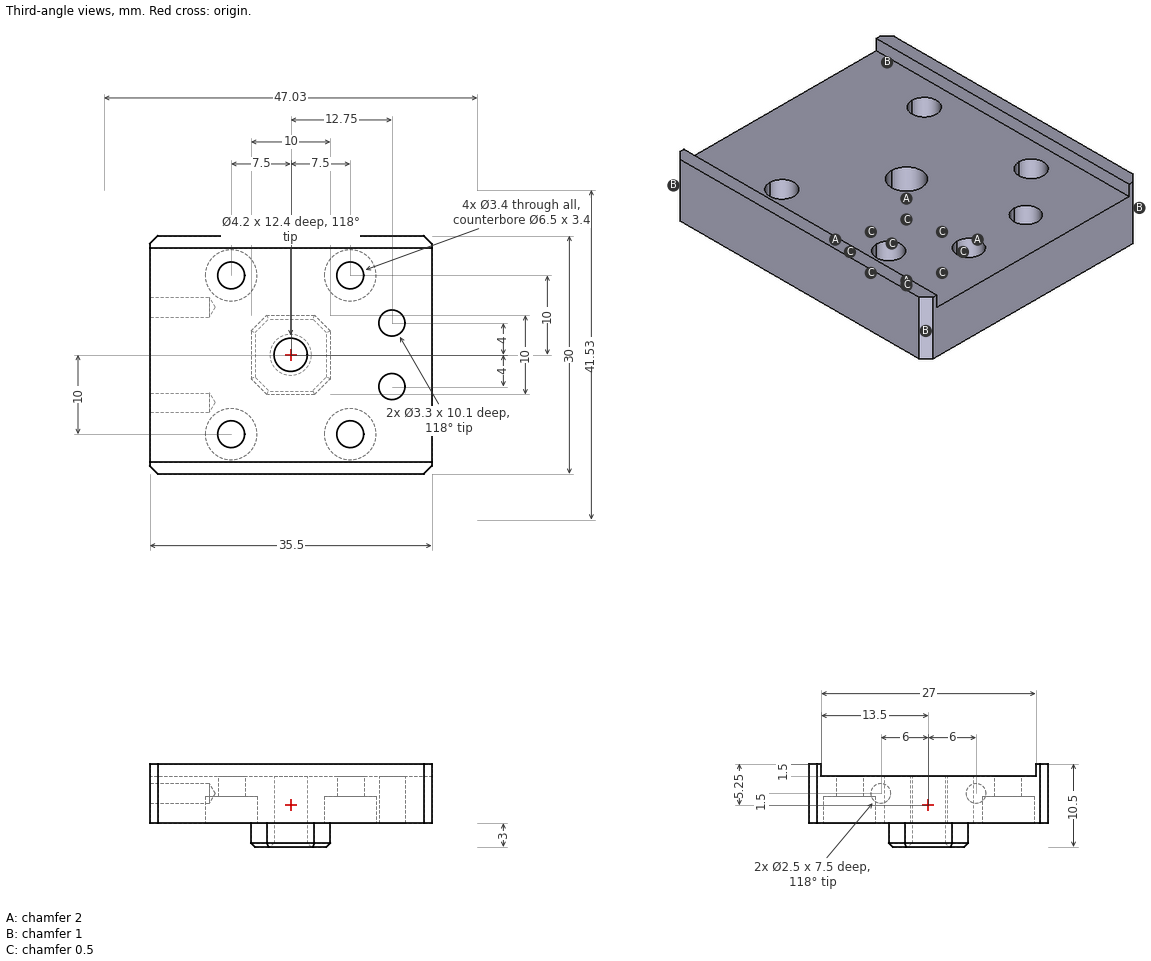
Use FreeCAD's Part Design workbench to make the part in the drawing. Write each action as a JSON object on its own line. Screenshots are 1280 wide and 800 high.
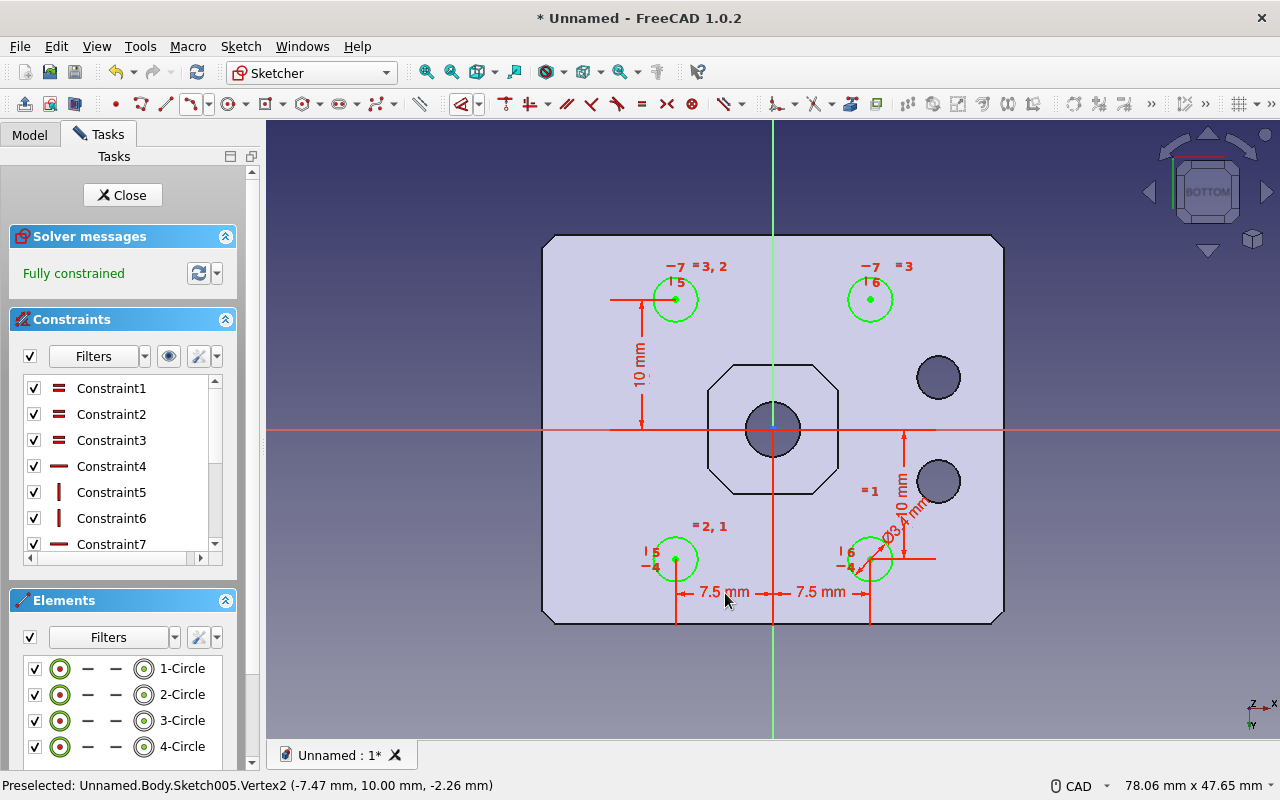
{"action": "left_click", "coordinate": [123, 195]}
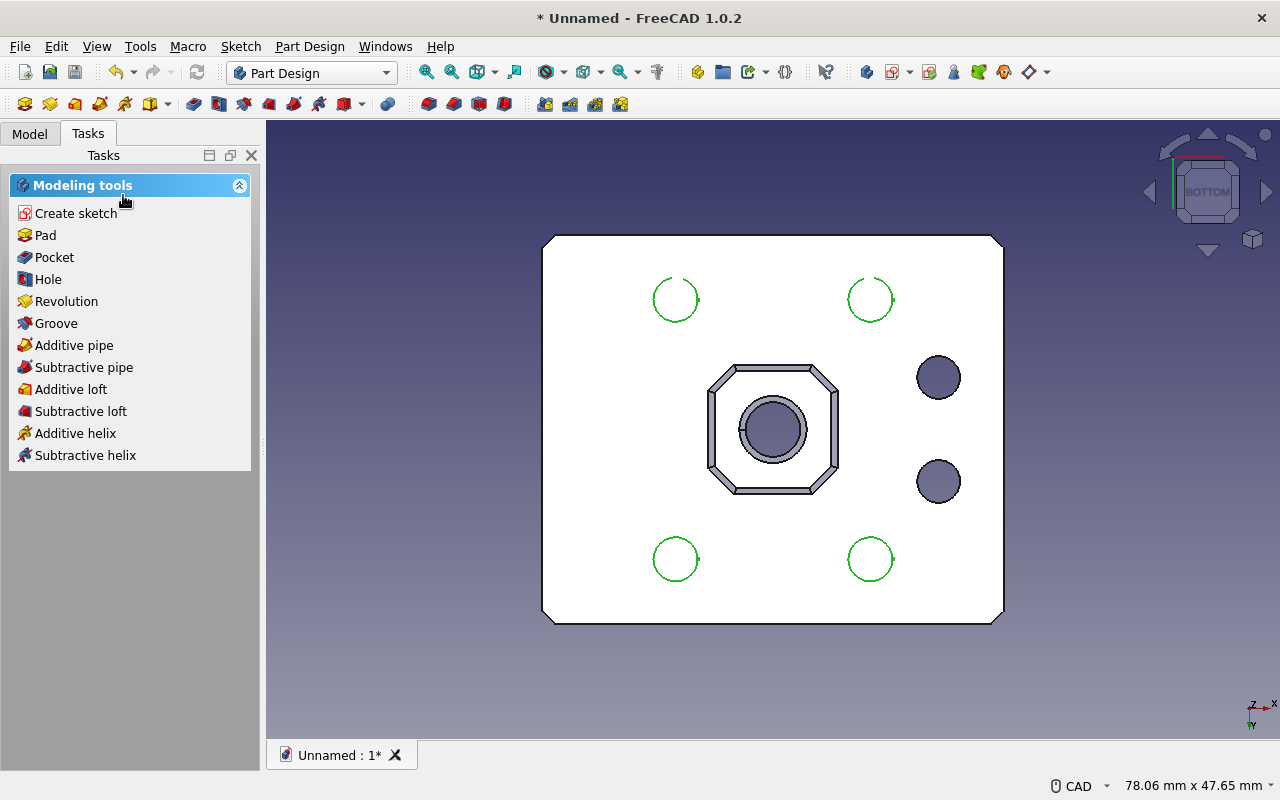
{"action": "left_click", "coordinate": [219, 104]}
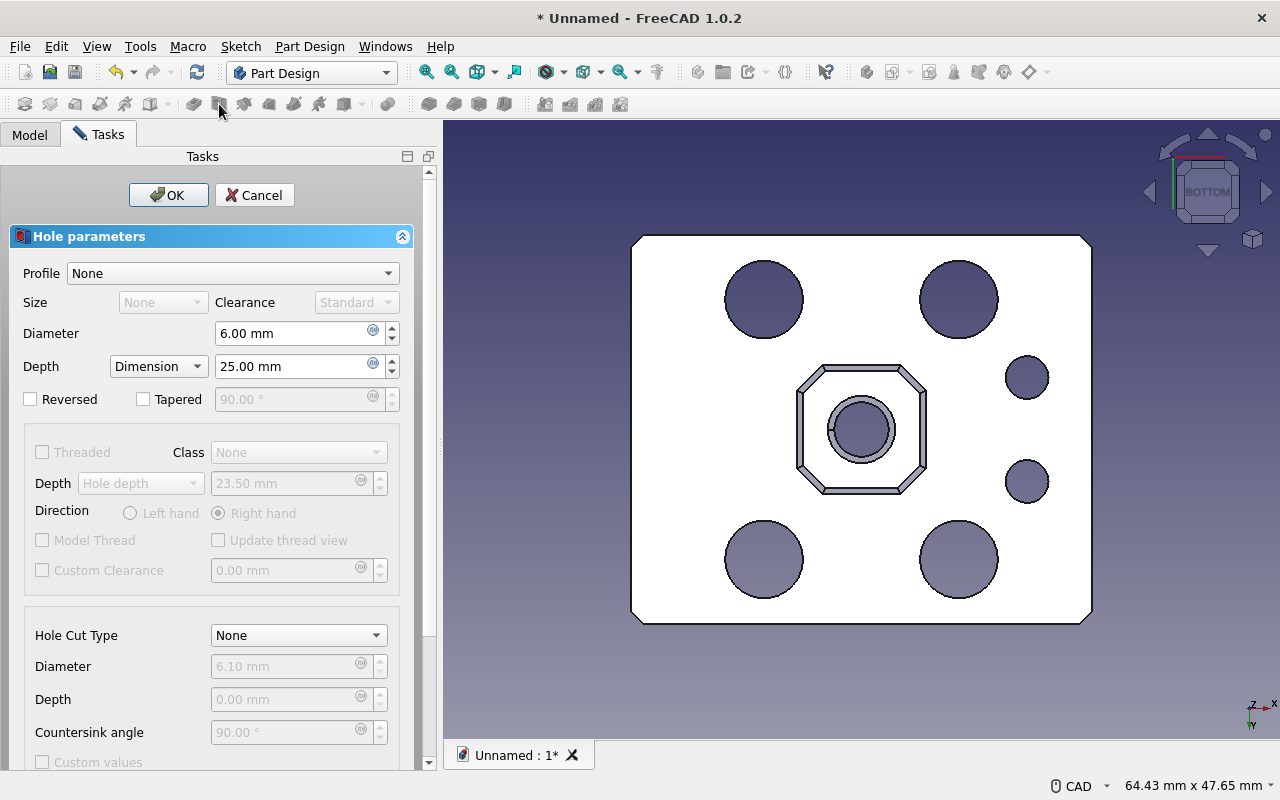
{"action": "triple_click", "coordinate": [300, 334]}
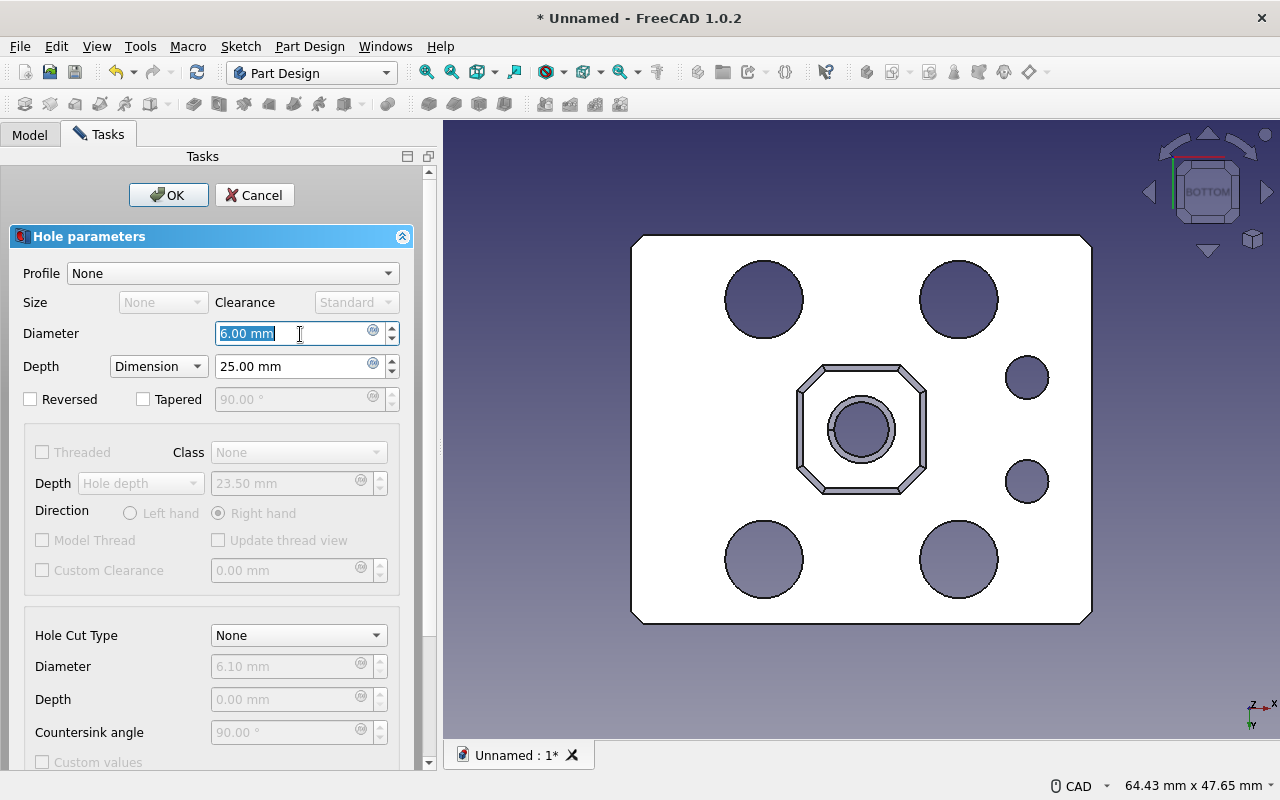
{"action": "type", "text": "3.4"}
{"action": "key", "text": "Tab"}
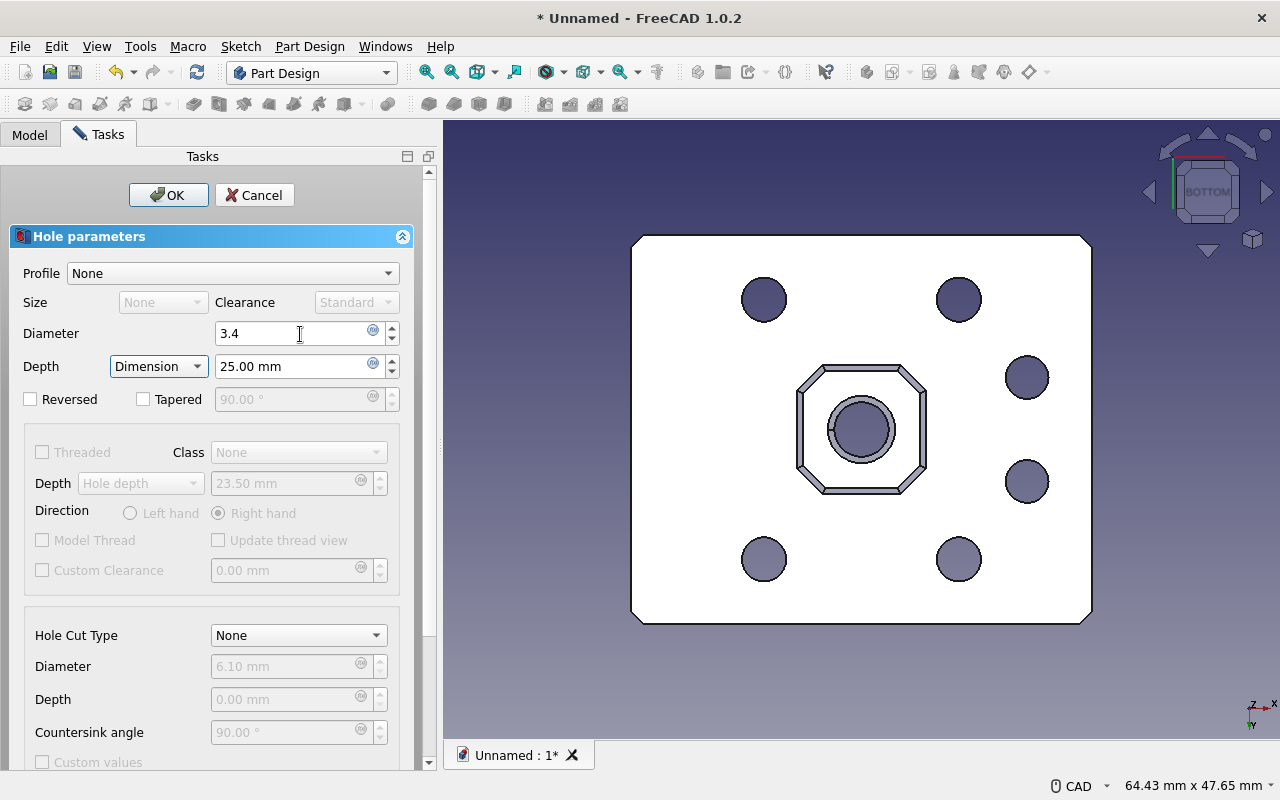
{"action": "left_click", "coordinate": [160, 366]}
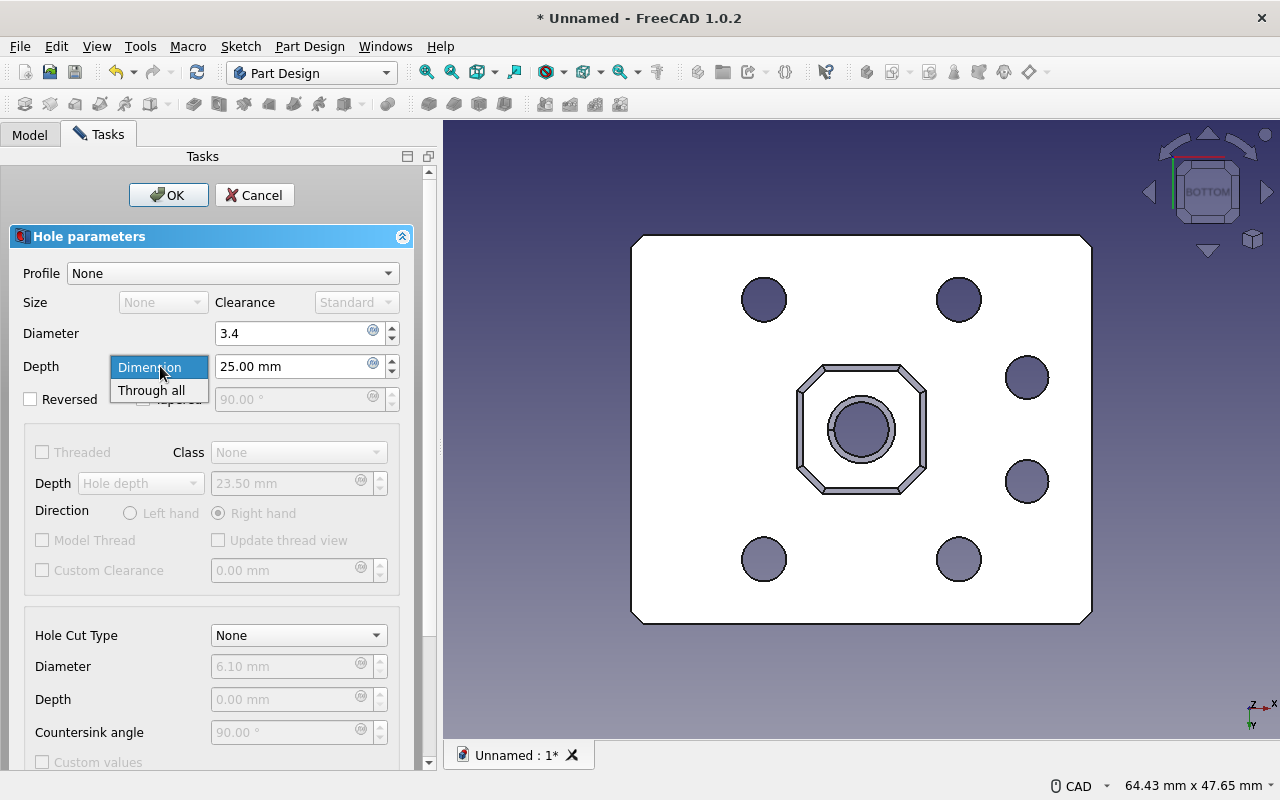
{"action": "left_click", "coordinate": [158, 390]}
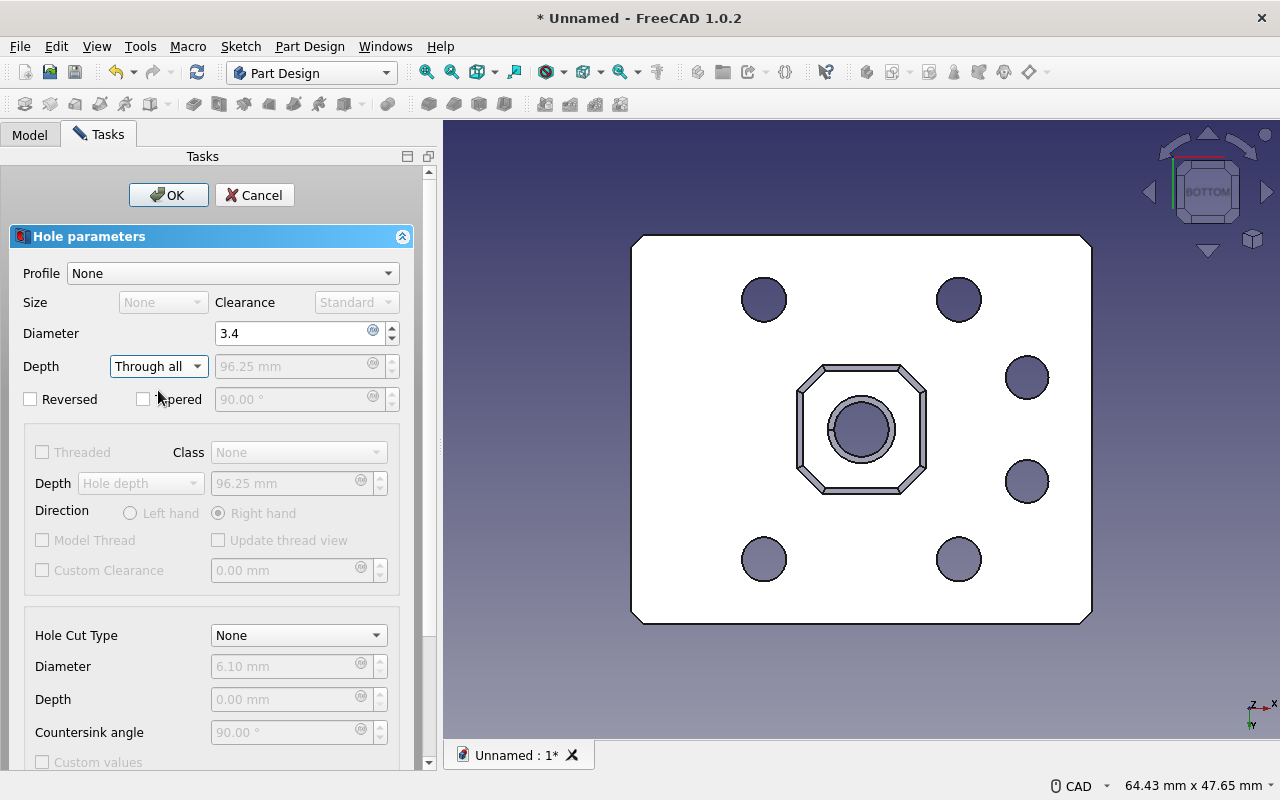
{"action": "left_click", "coordinate": [300, 636]}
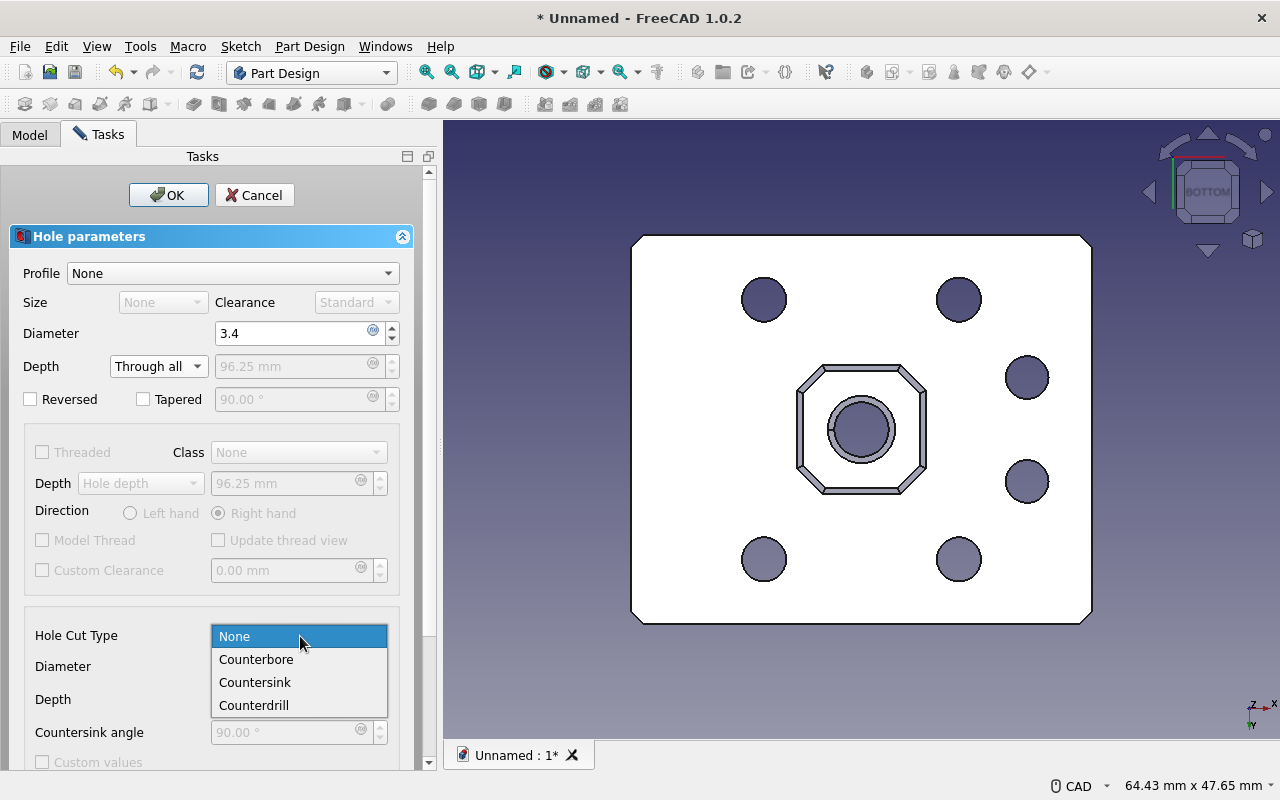
{"action": "left_click", "coordinate": [298, 660]}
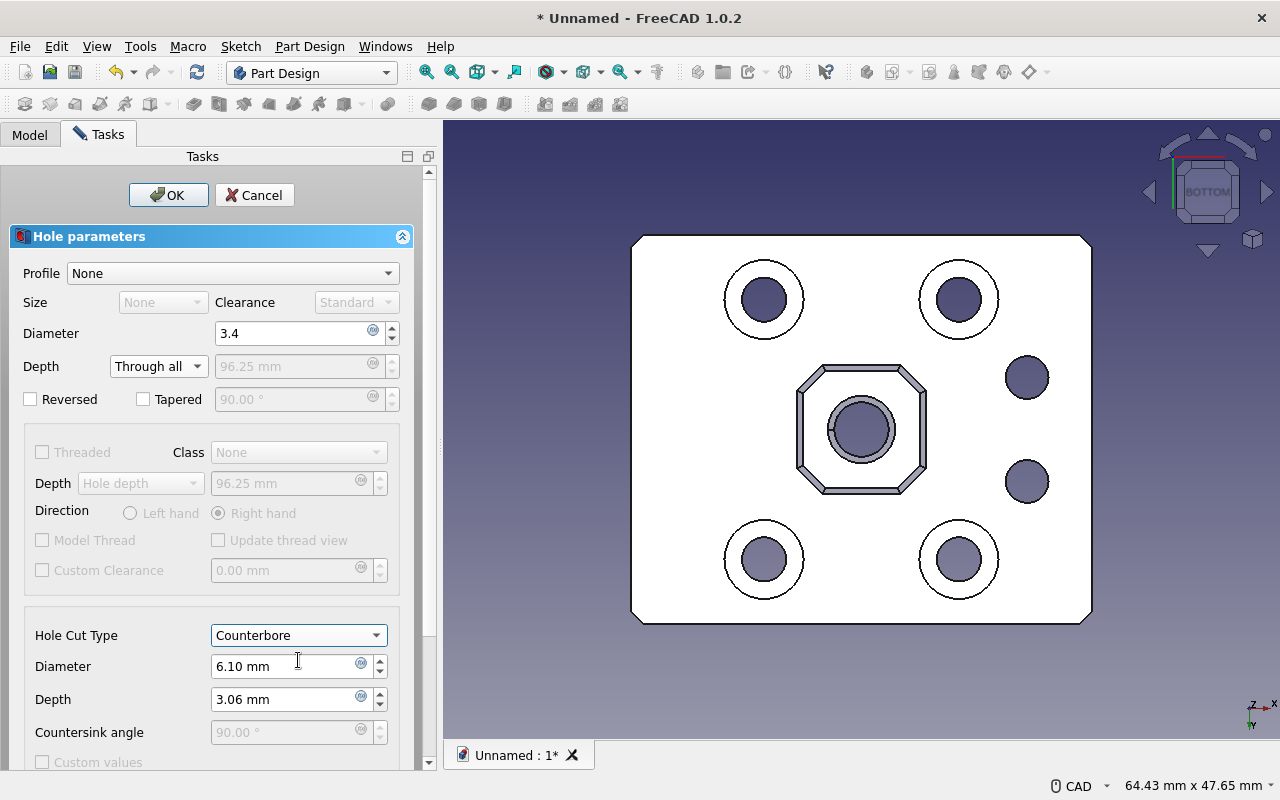
{"action": "triple_click", "coordinate": [292, 666]}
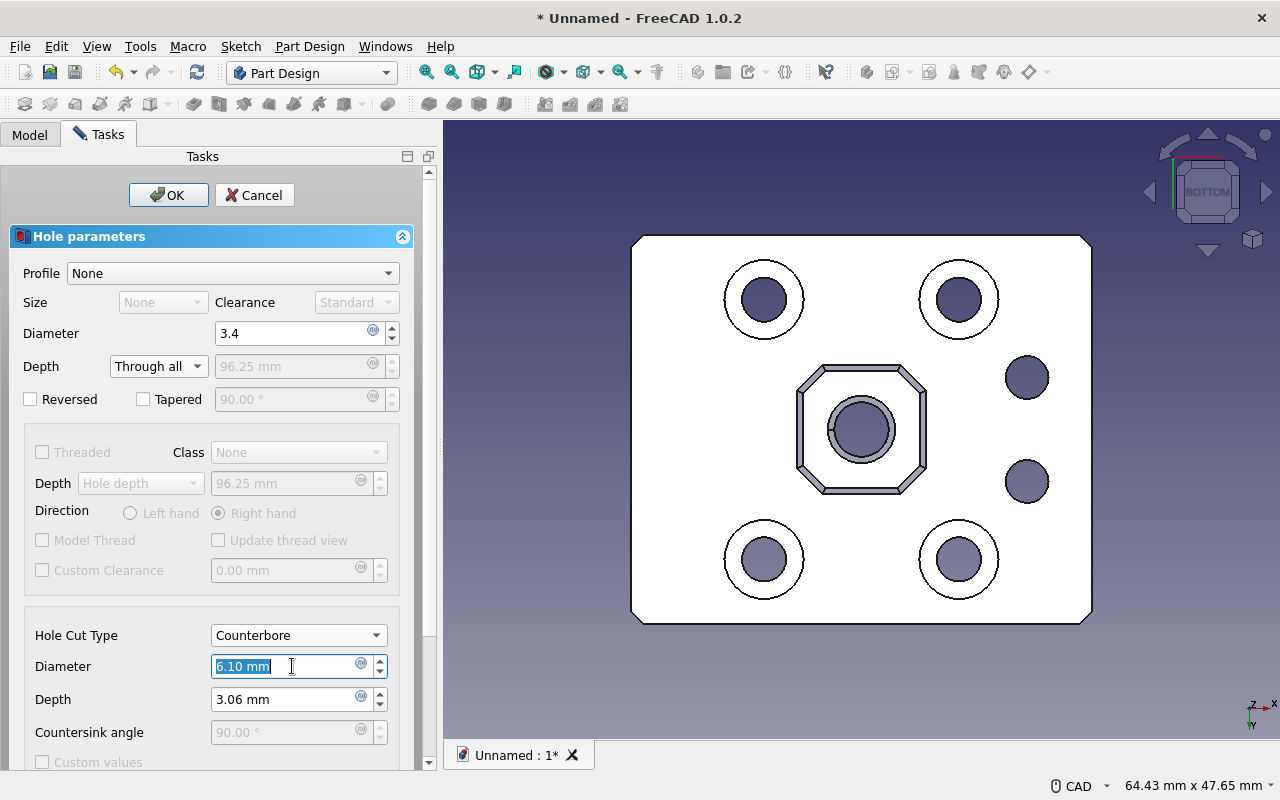
{"action": "type", "text": "6.5"}
{"action": "key", "text": "Tab"}